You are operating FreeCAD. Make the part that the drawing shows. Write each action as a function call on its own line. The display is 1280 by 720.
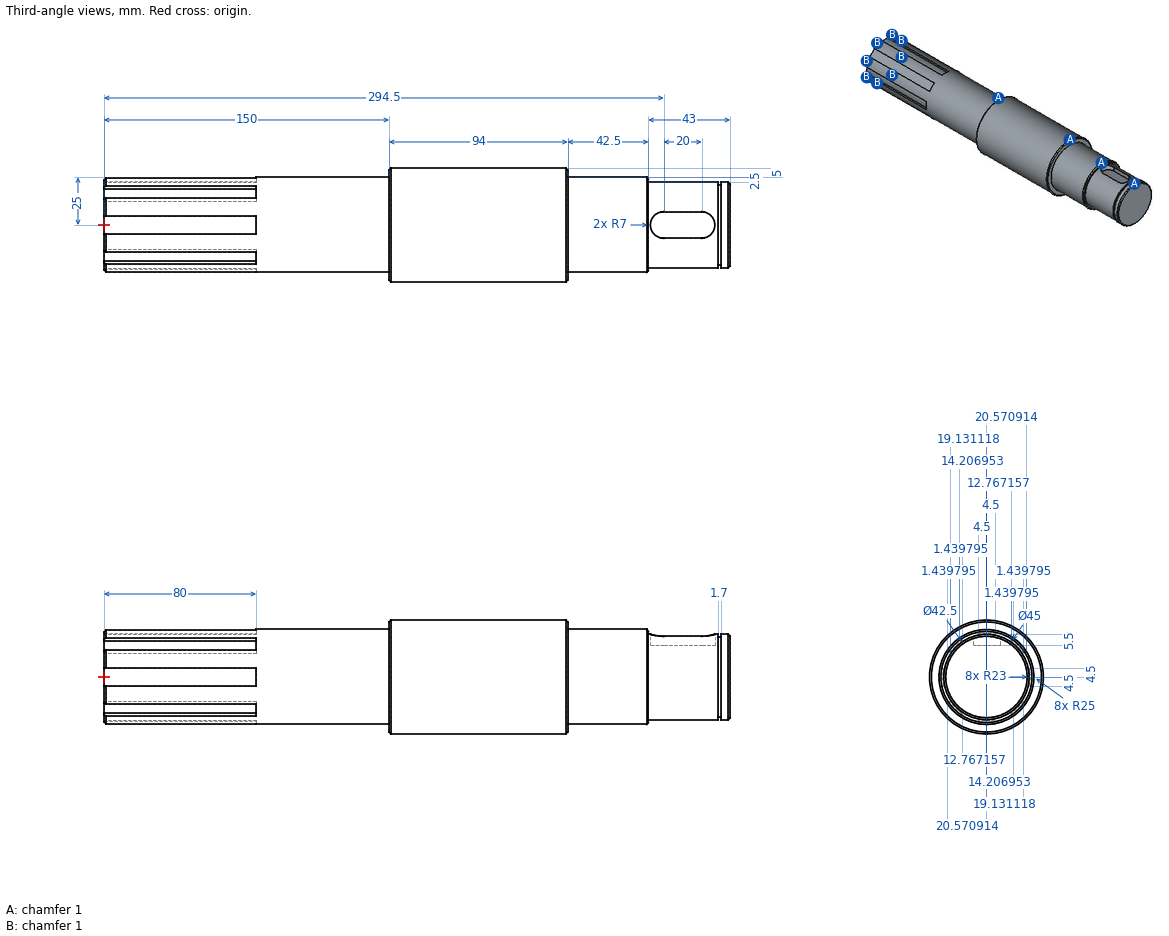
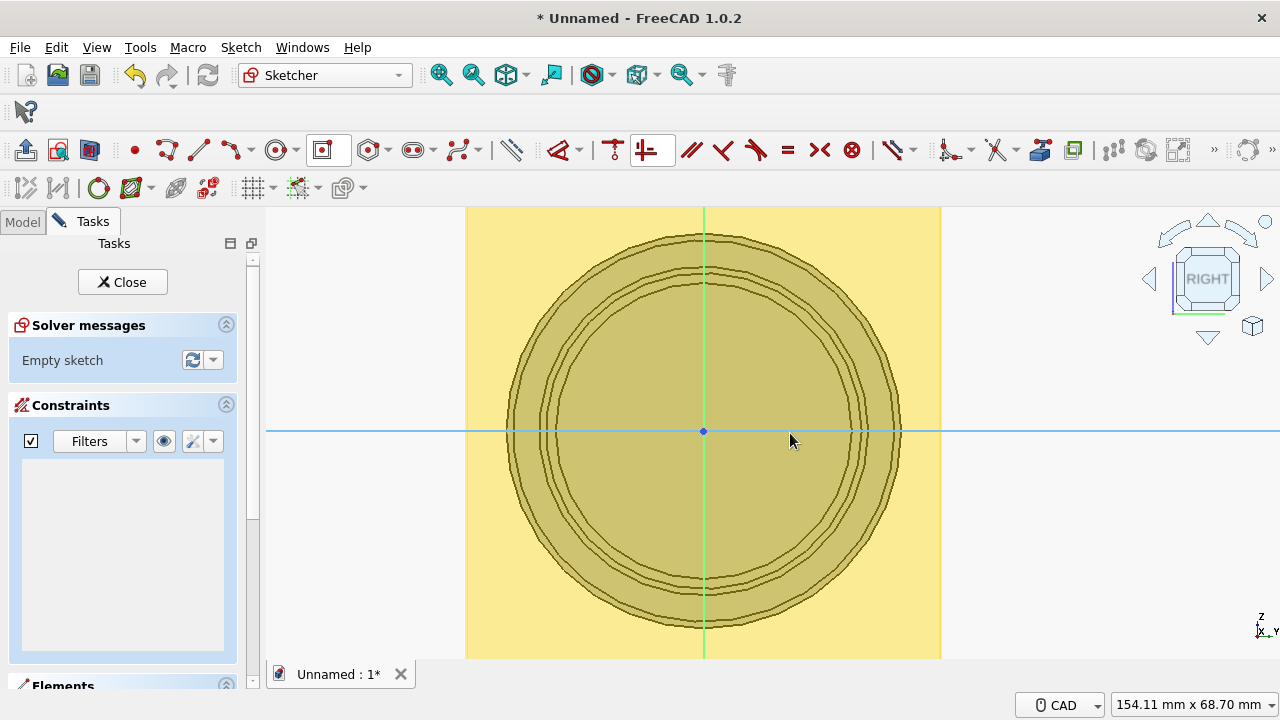
click(276, 150)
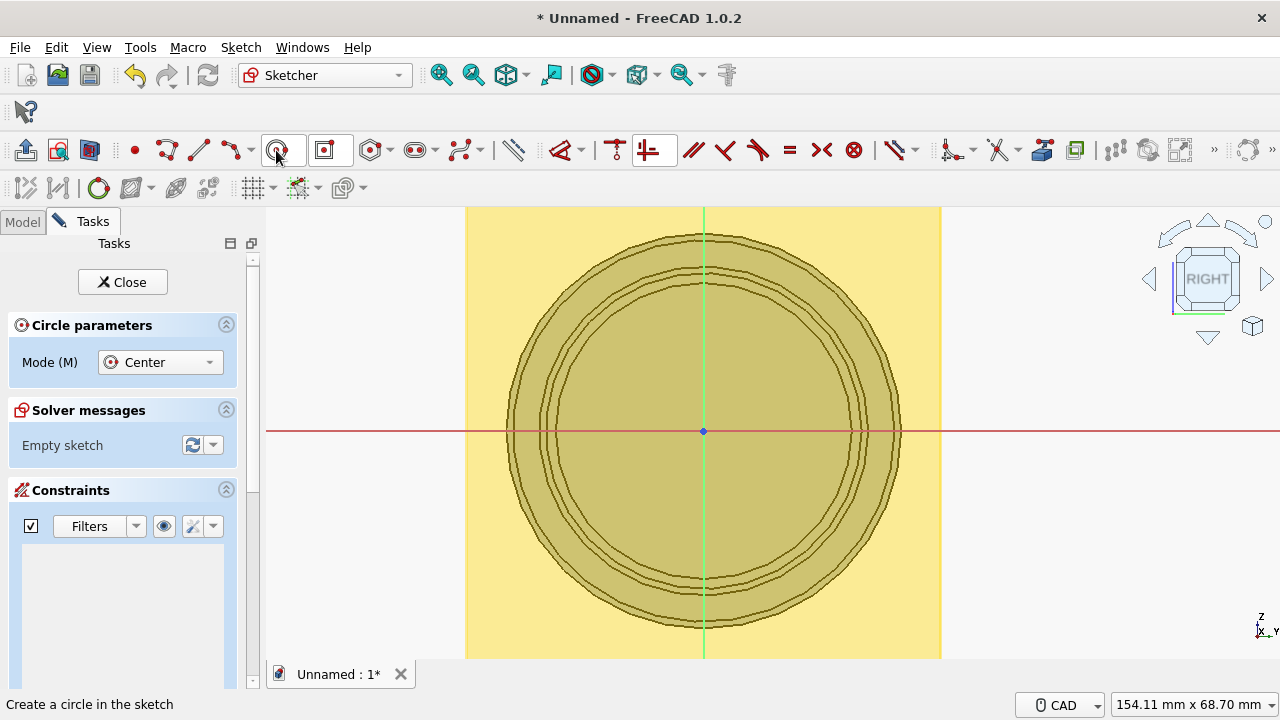
click(704, 431)
click(808, 326)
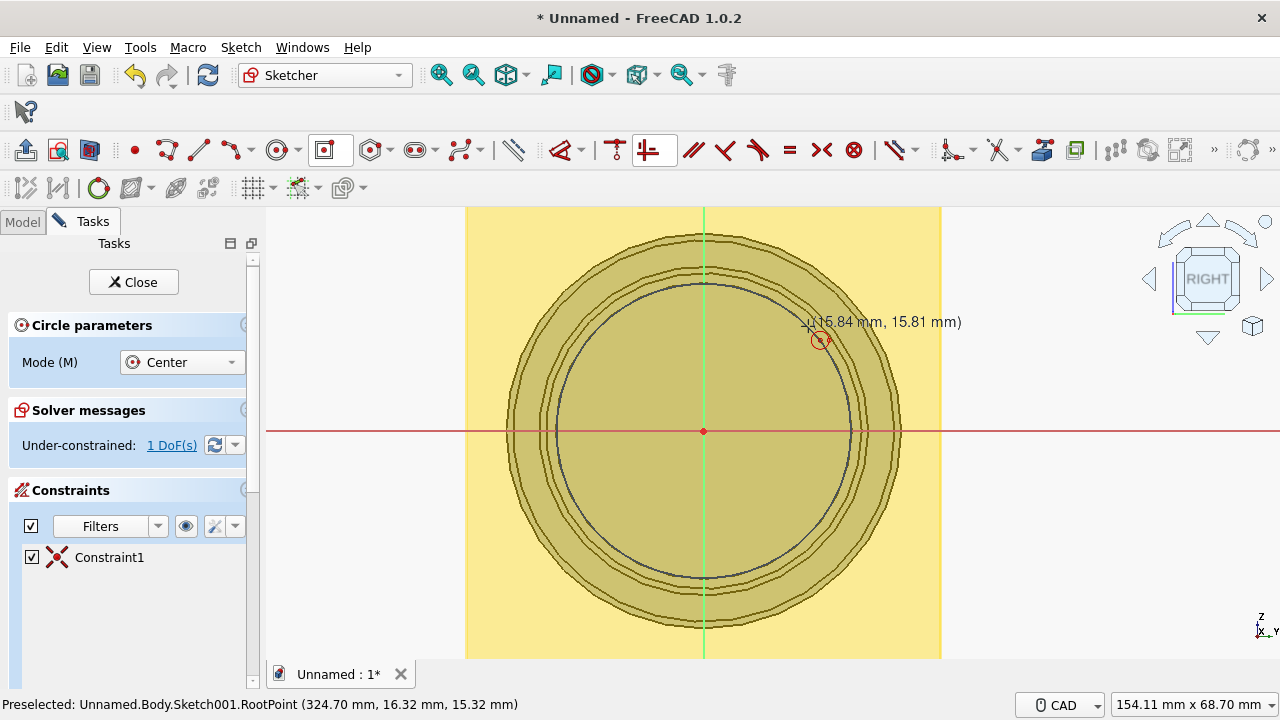
click(704, 431)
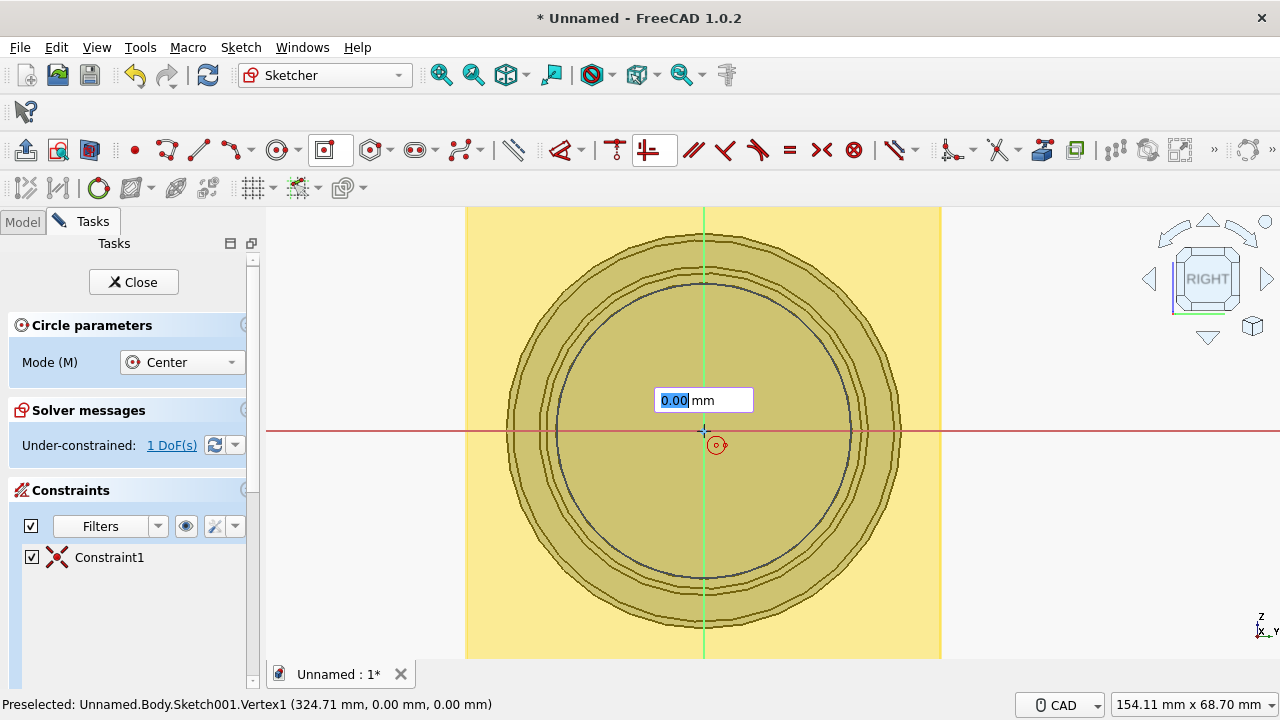
scroll(803, 332, up, 4)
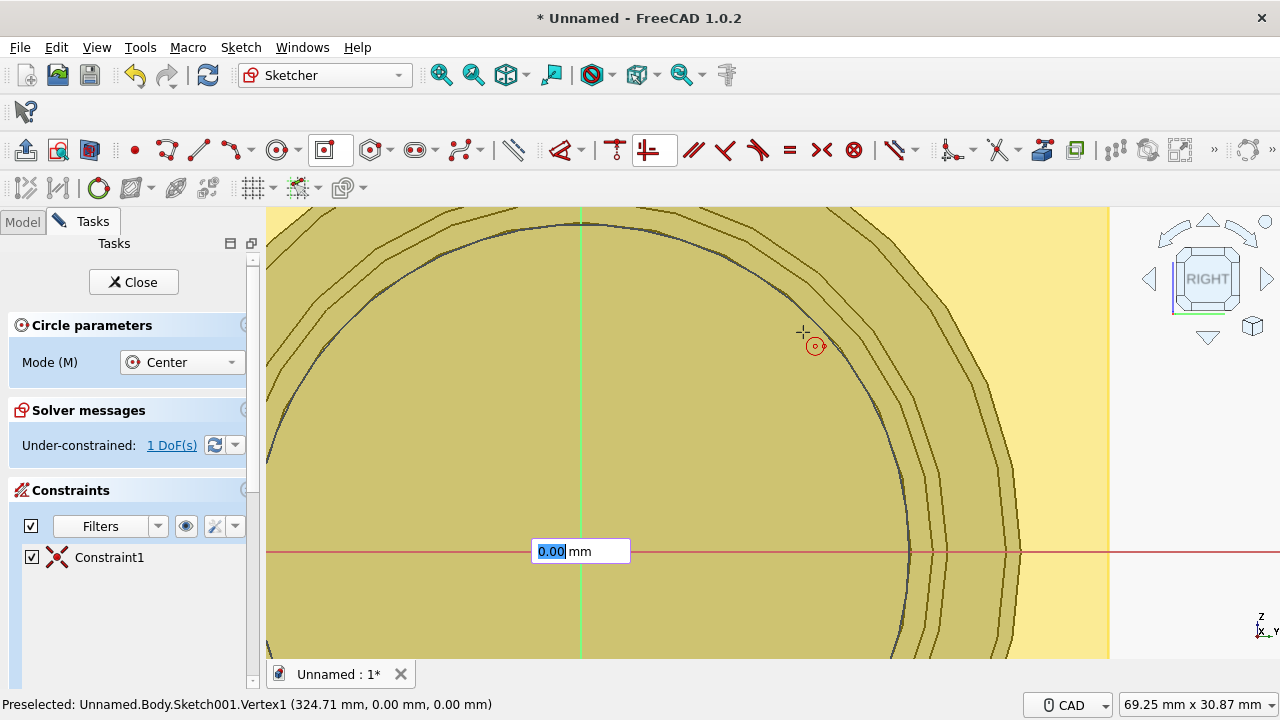
click(802, 332)
key(Escape)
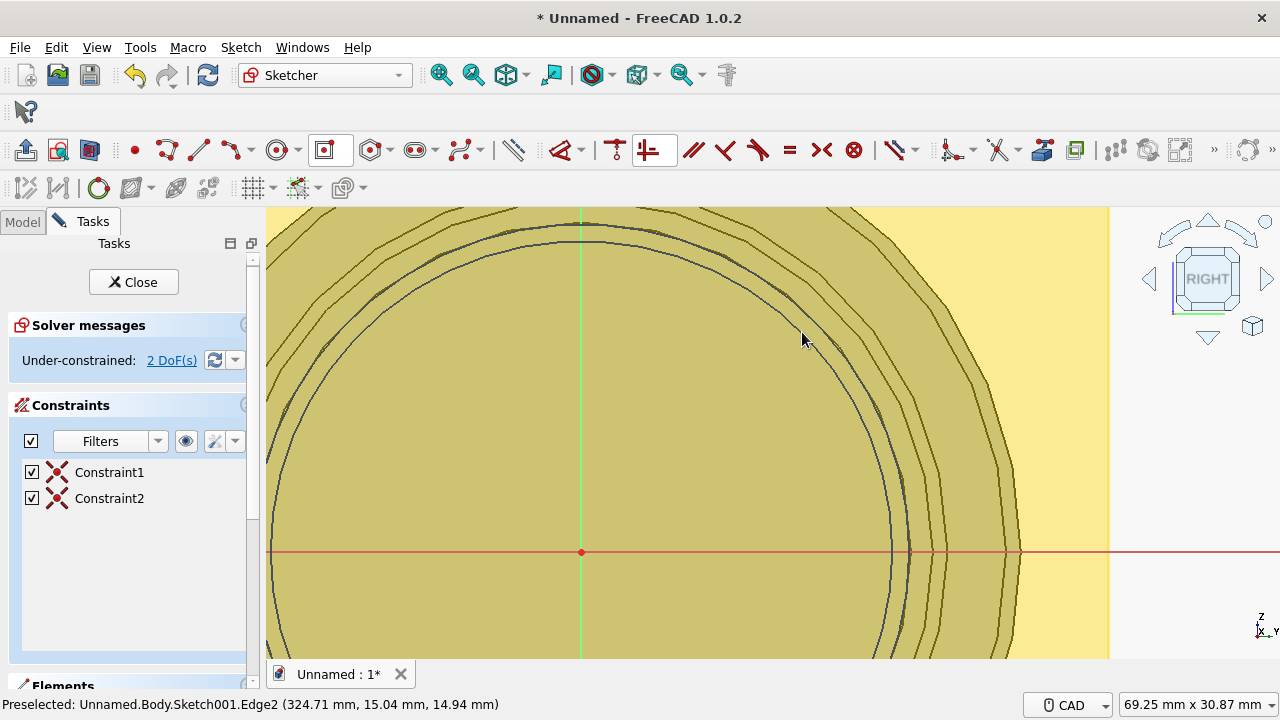
click(560, 150)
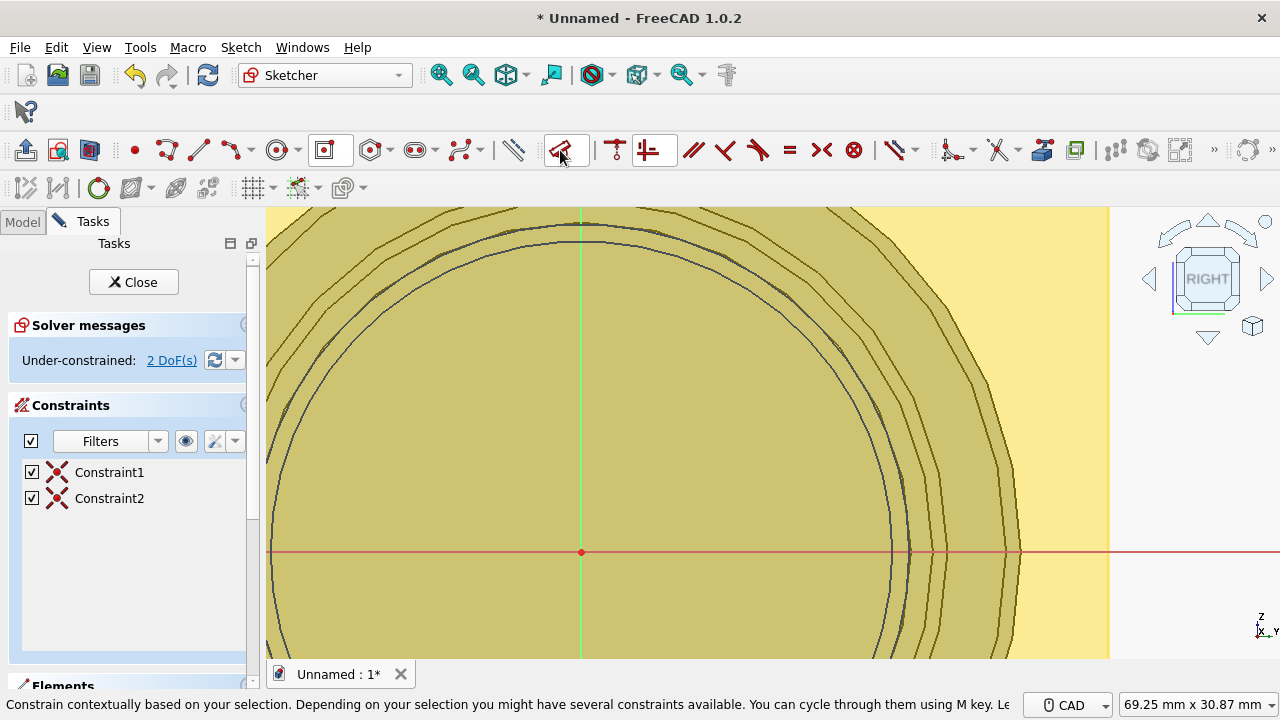
click(813, 320)
click(836, 297)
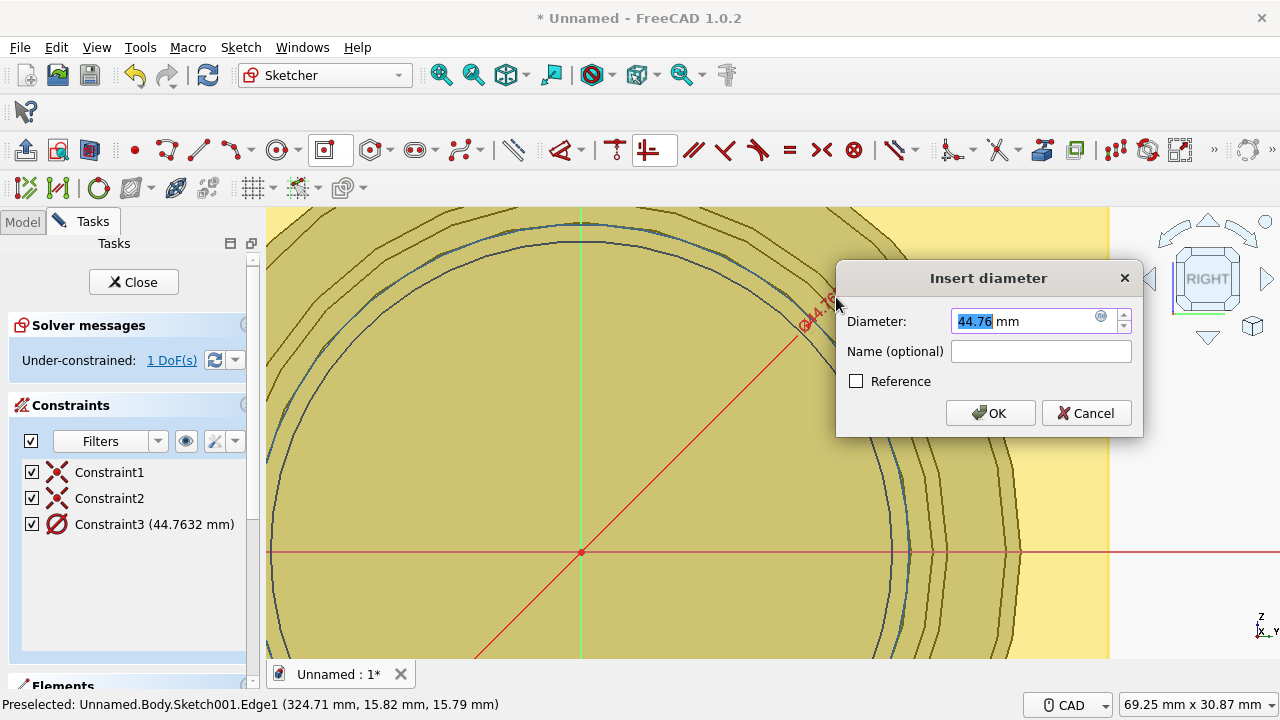
text(45)
key(Return)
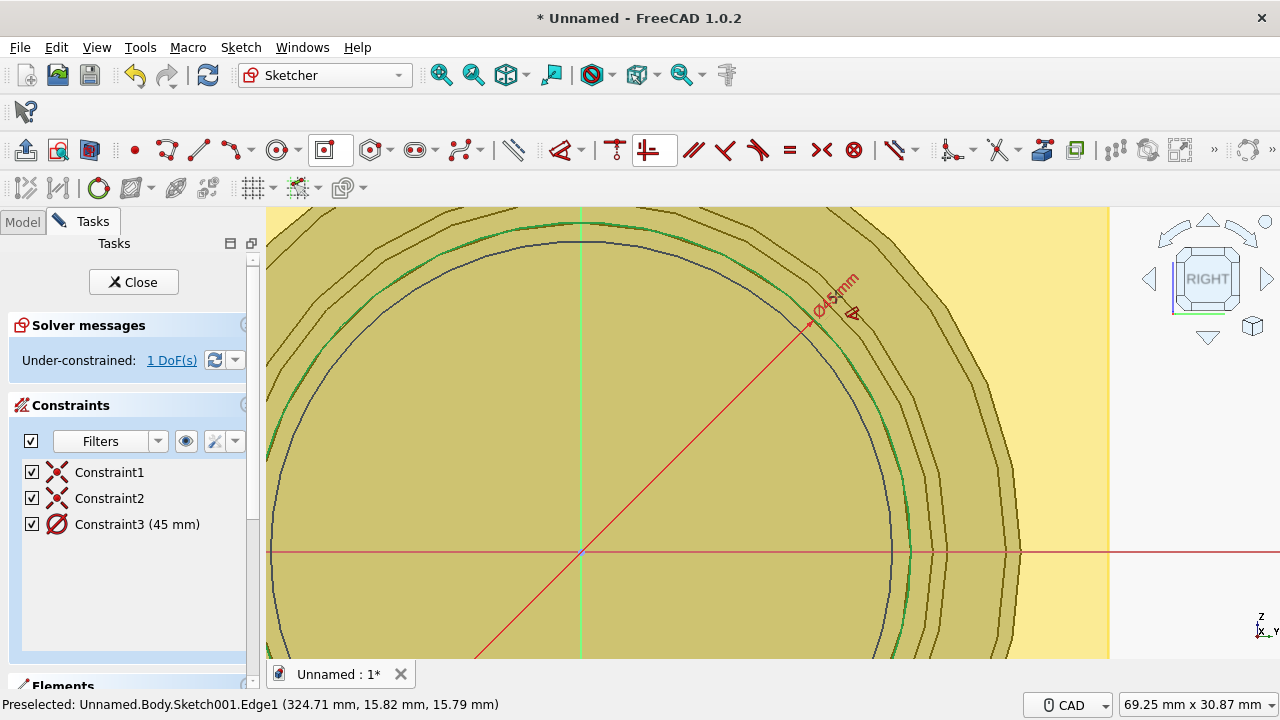
click(801, 332)
click(910, 455)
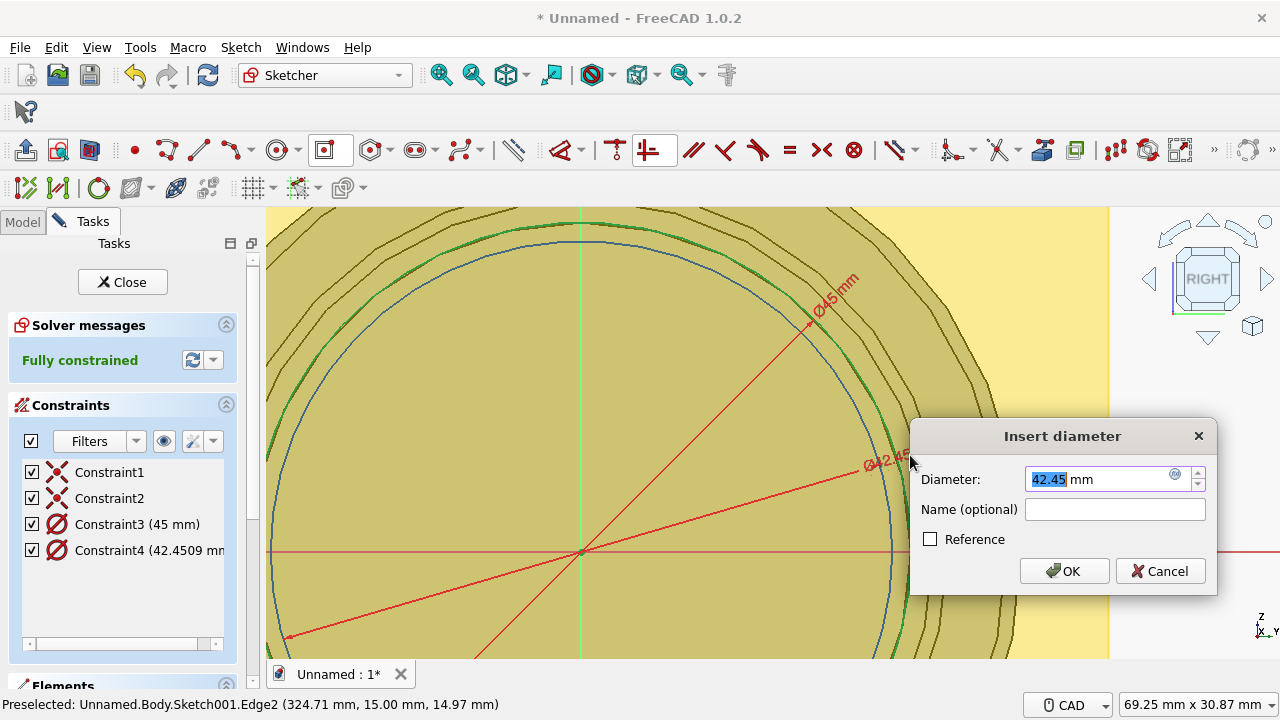
text(42.5)
key(Return)
key(Escape)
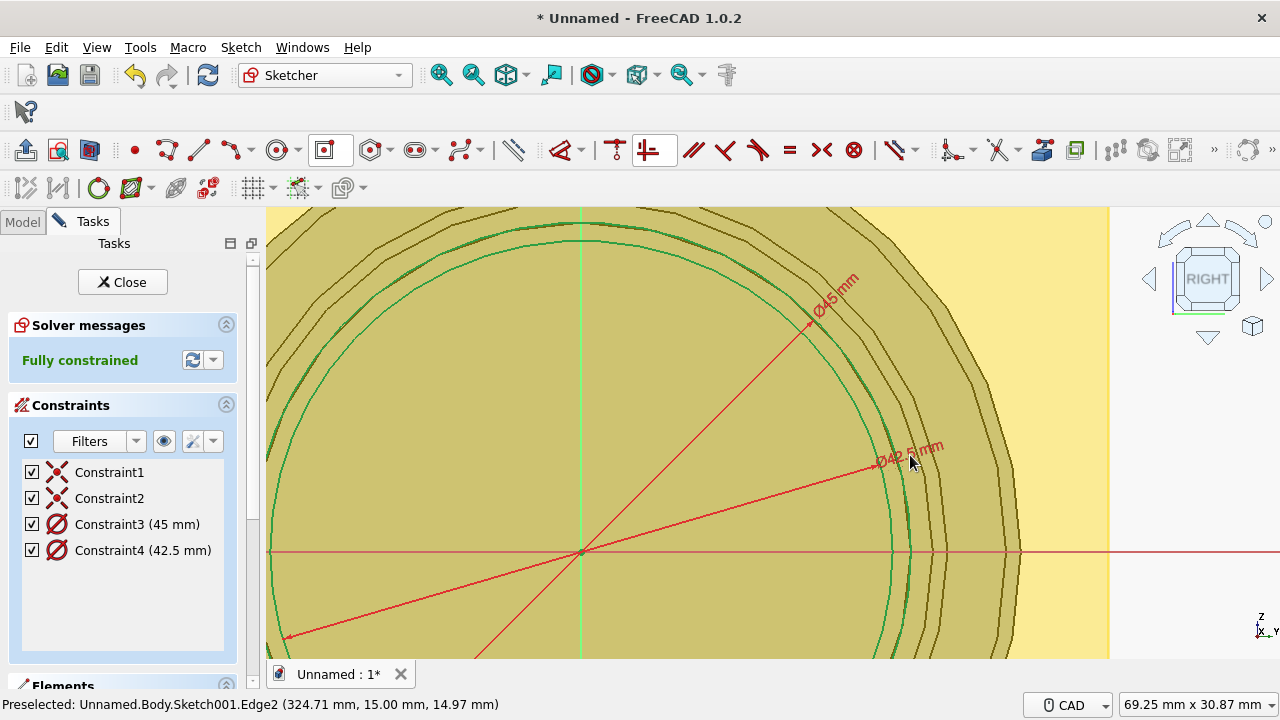
click(123, 282)